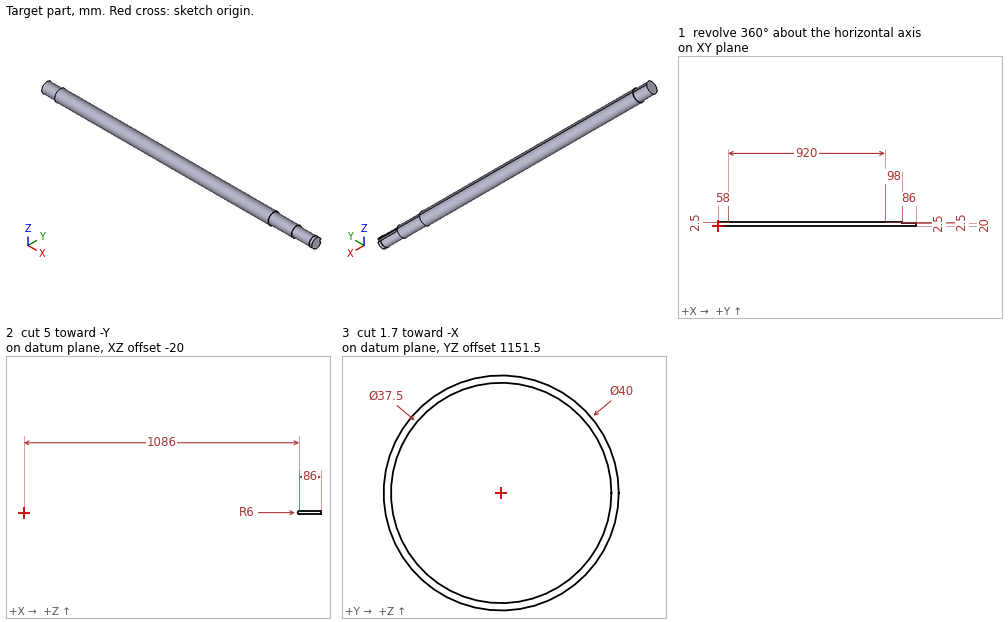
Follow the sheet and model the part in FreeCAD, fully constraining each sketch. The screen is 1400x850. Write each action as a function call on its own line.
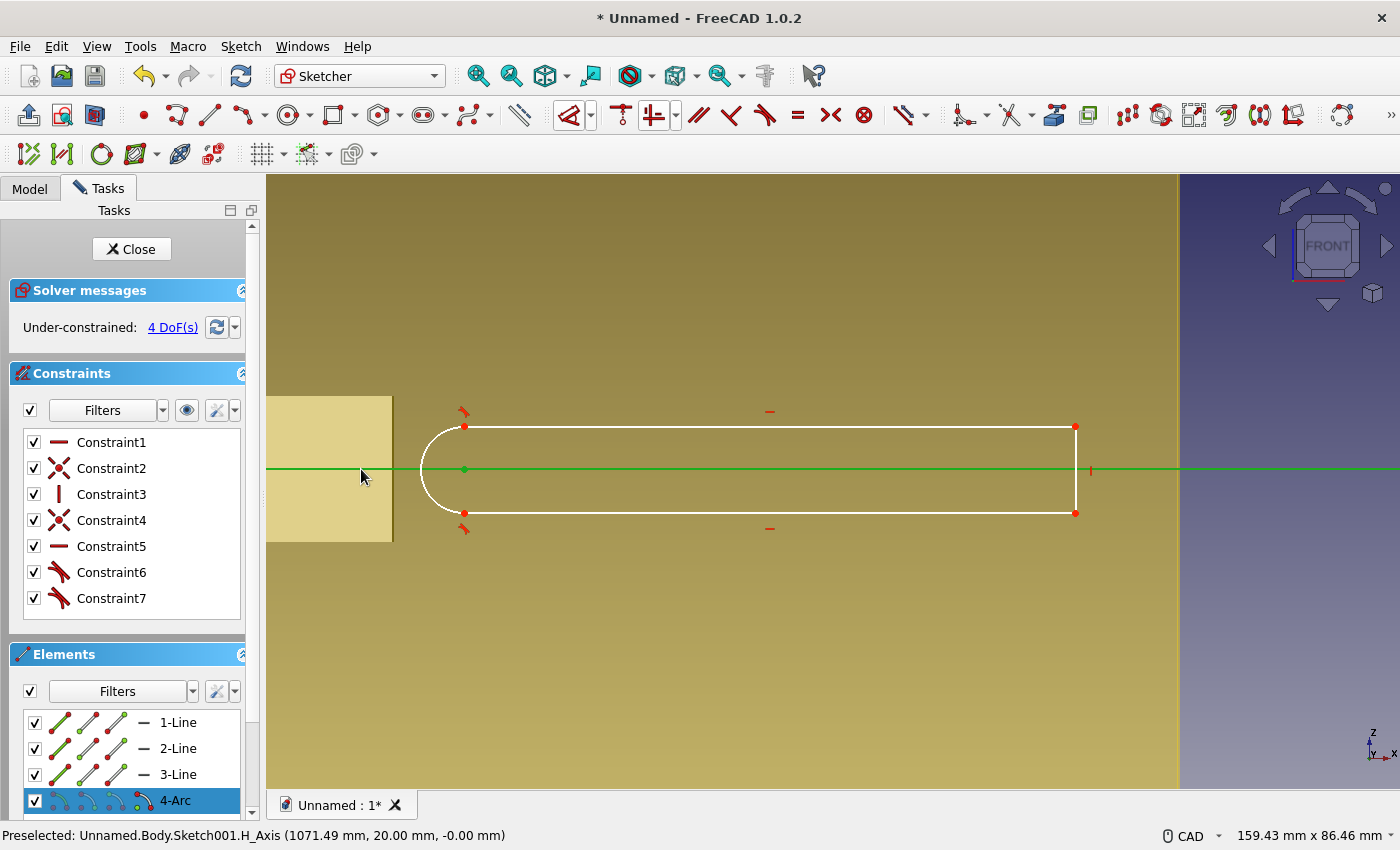
click(621, 116)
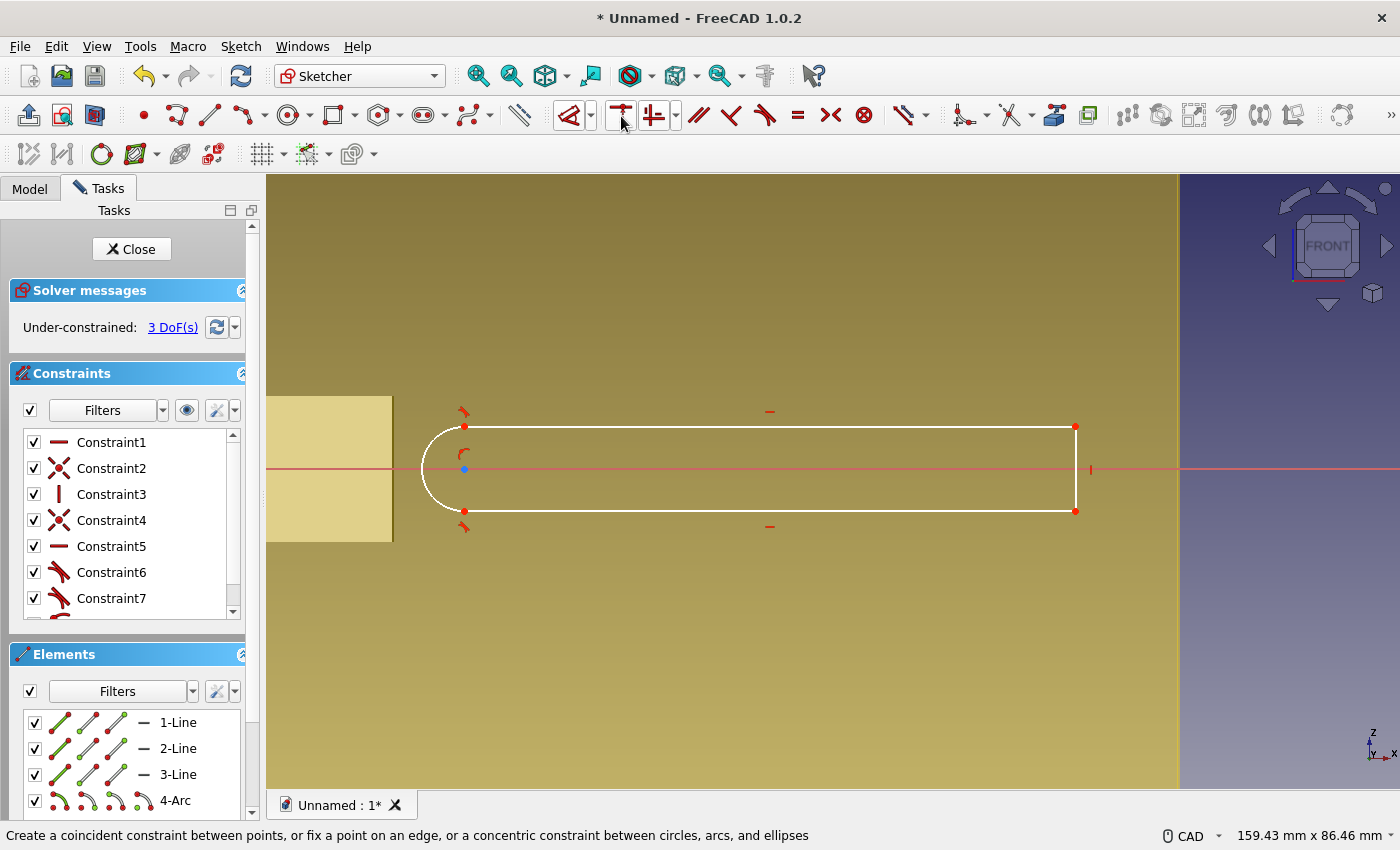
click(430, 444)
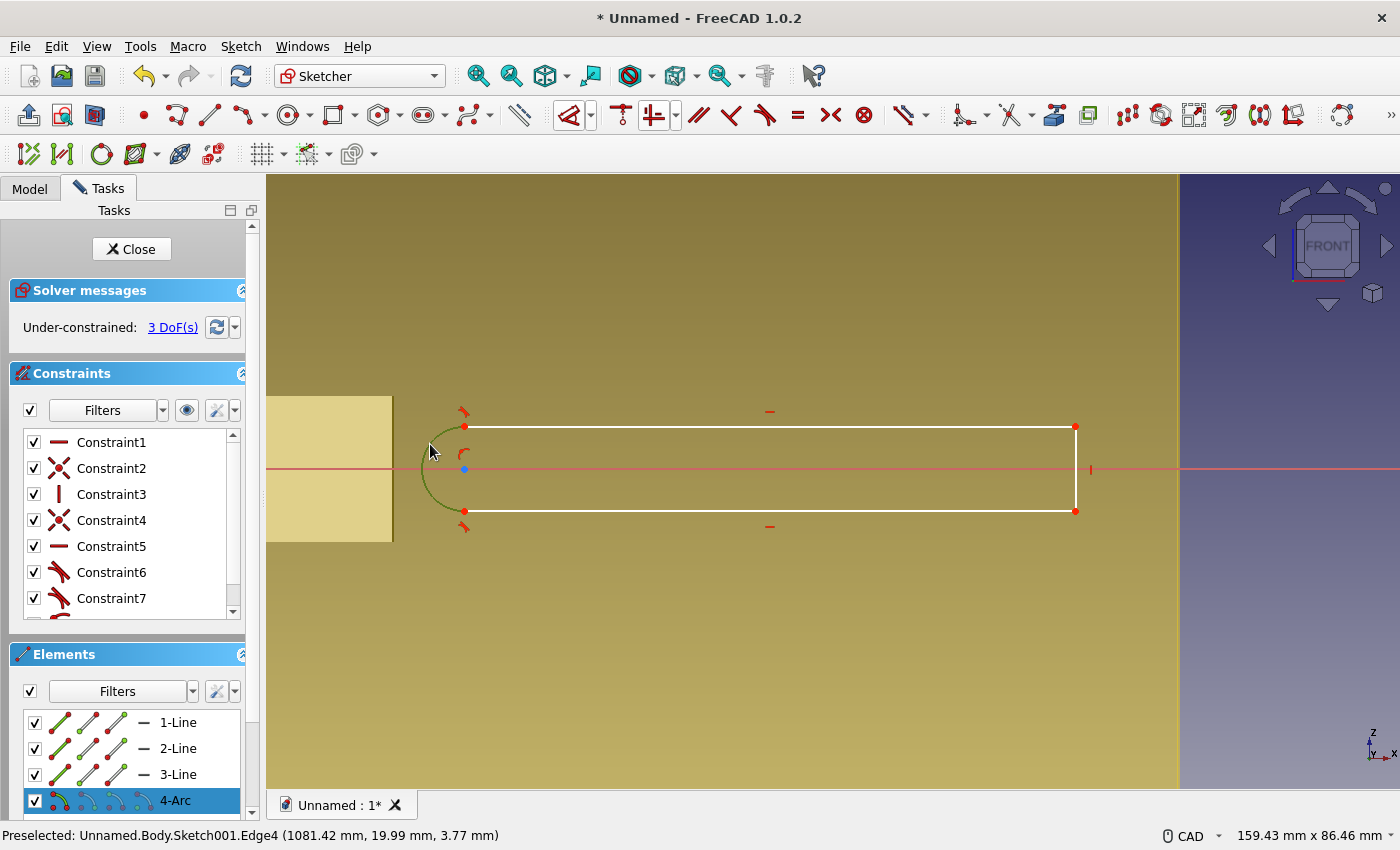
key(k)
key(r)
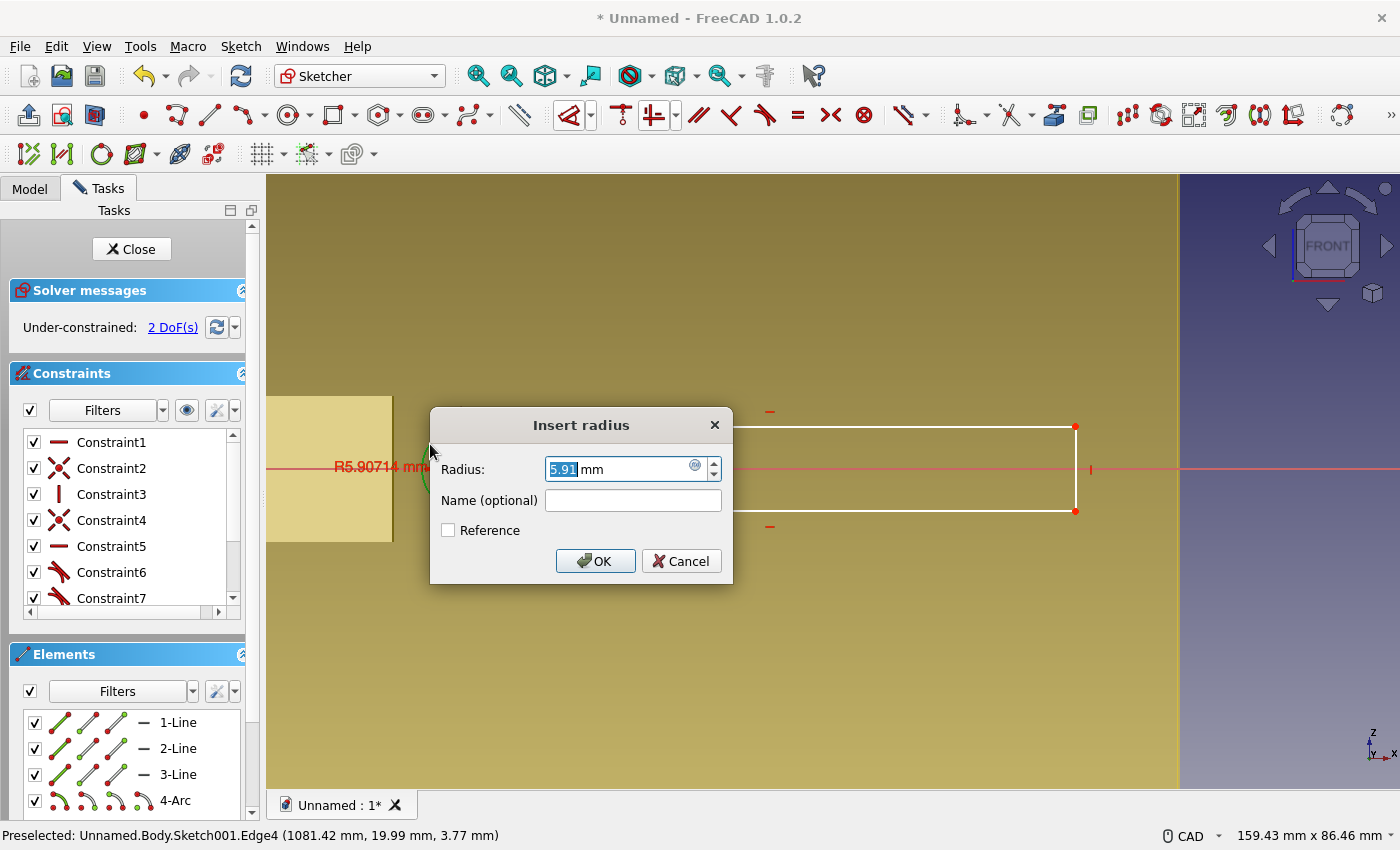
text(6)
key(Return)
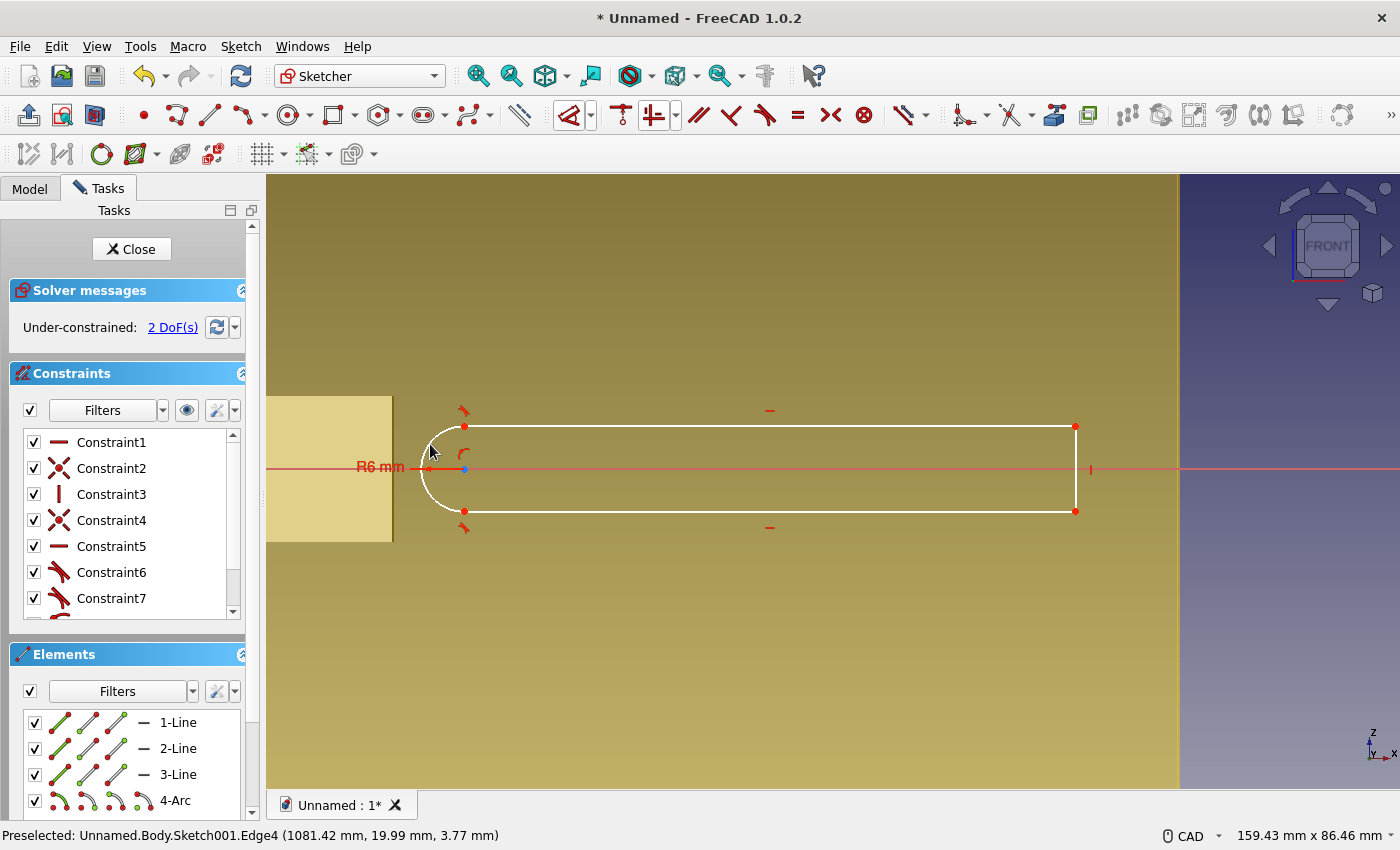
click(648, 426)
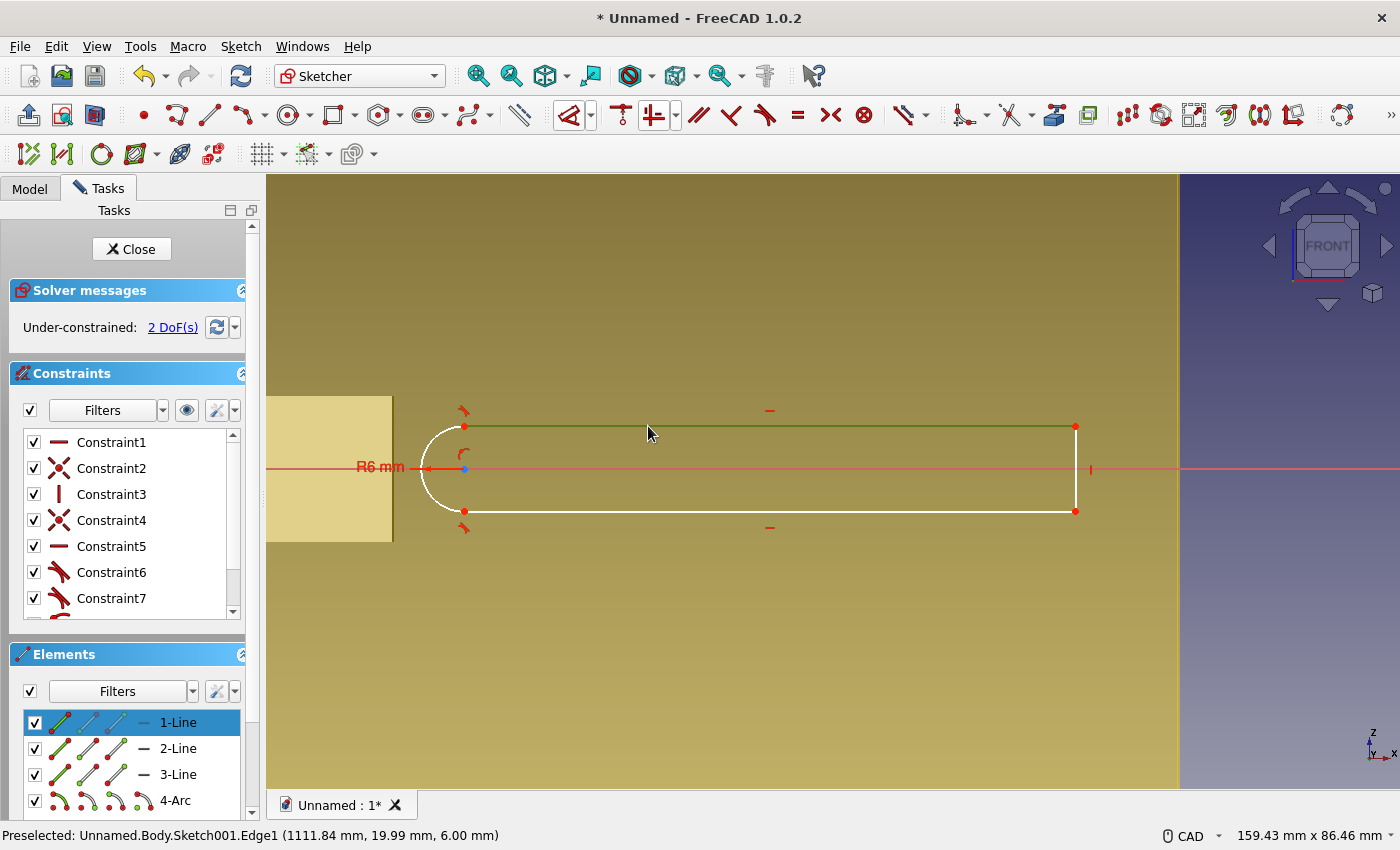
click(590, 116)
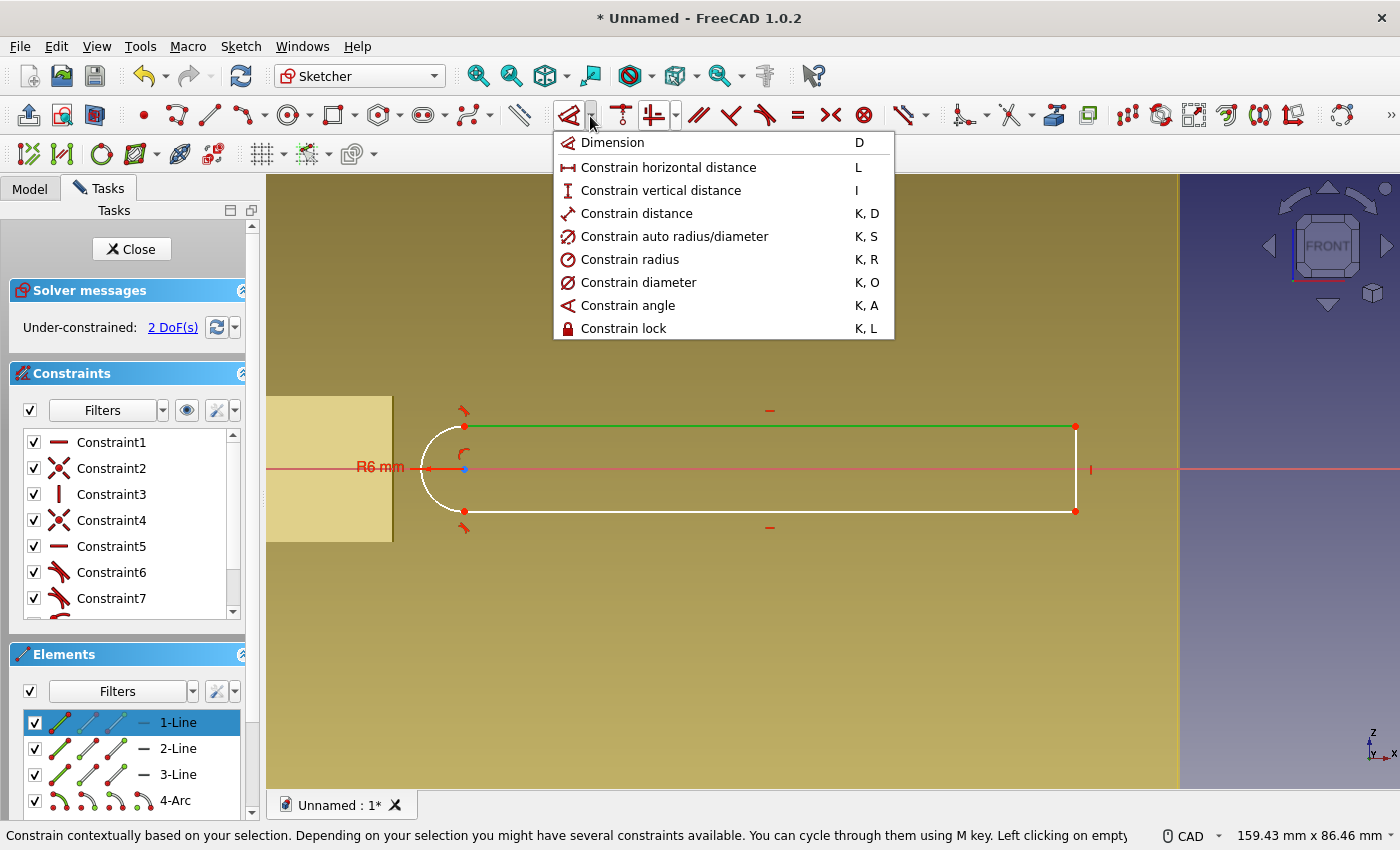
click(724, 168)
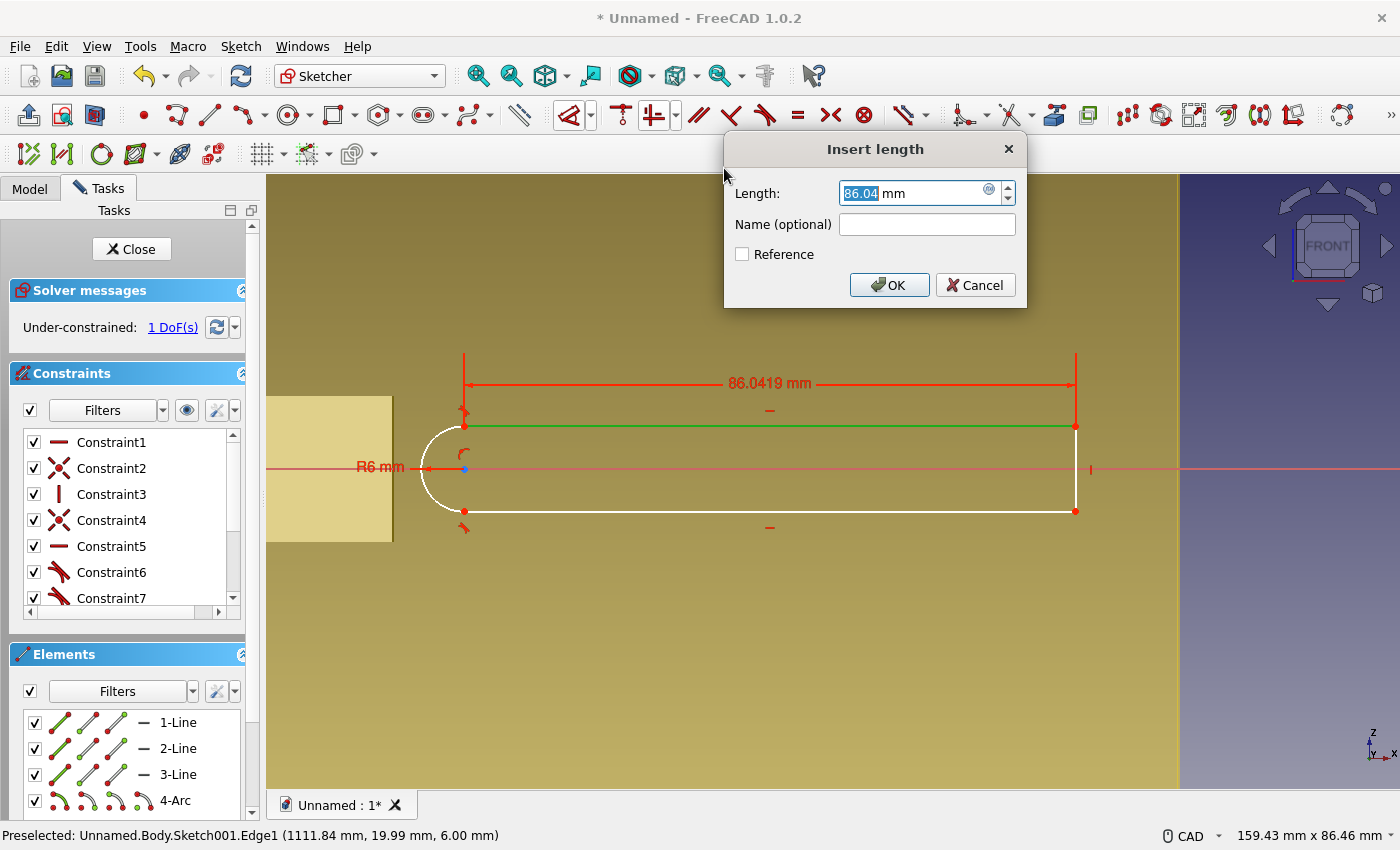
text(86)
key(Return)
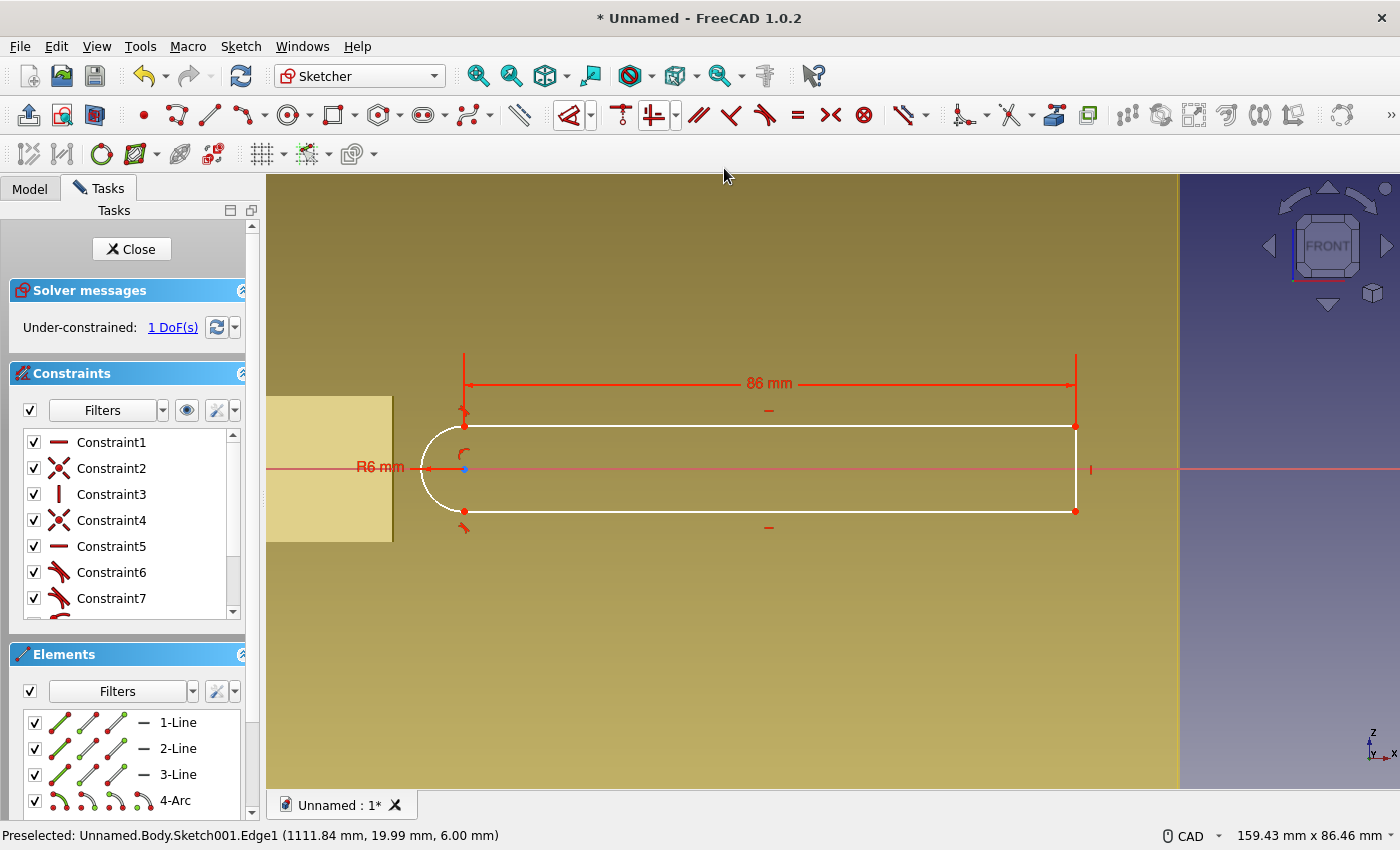
click(464, 426)